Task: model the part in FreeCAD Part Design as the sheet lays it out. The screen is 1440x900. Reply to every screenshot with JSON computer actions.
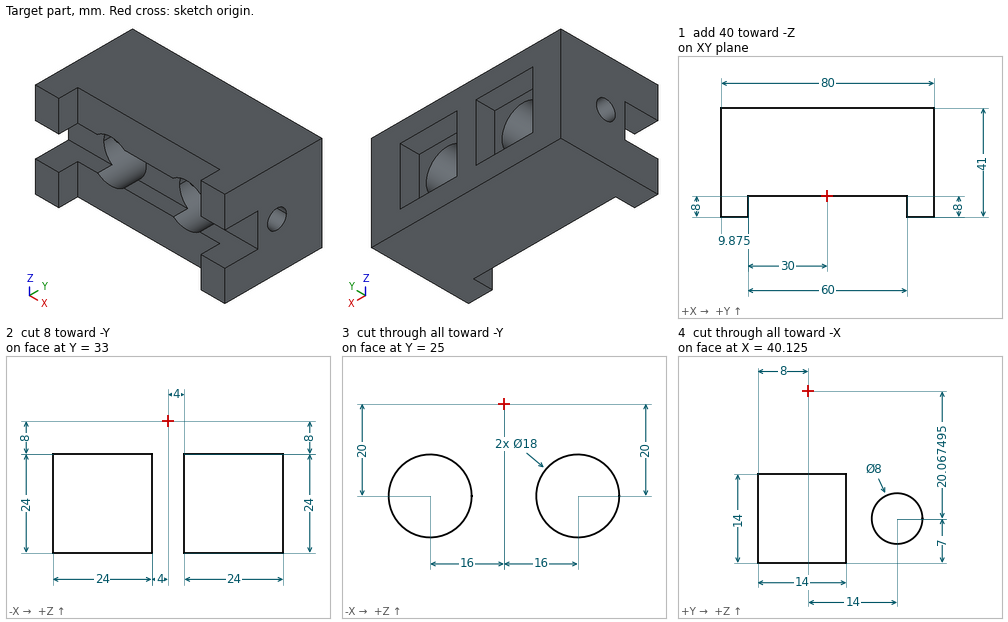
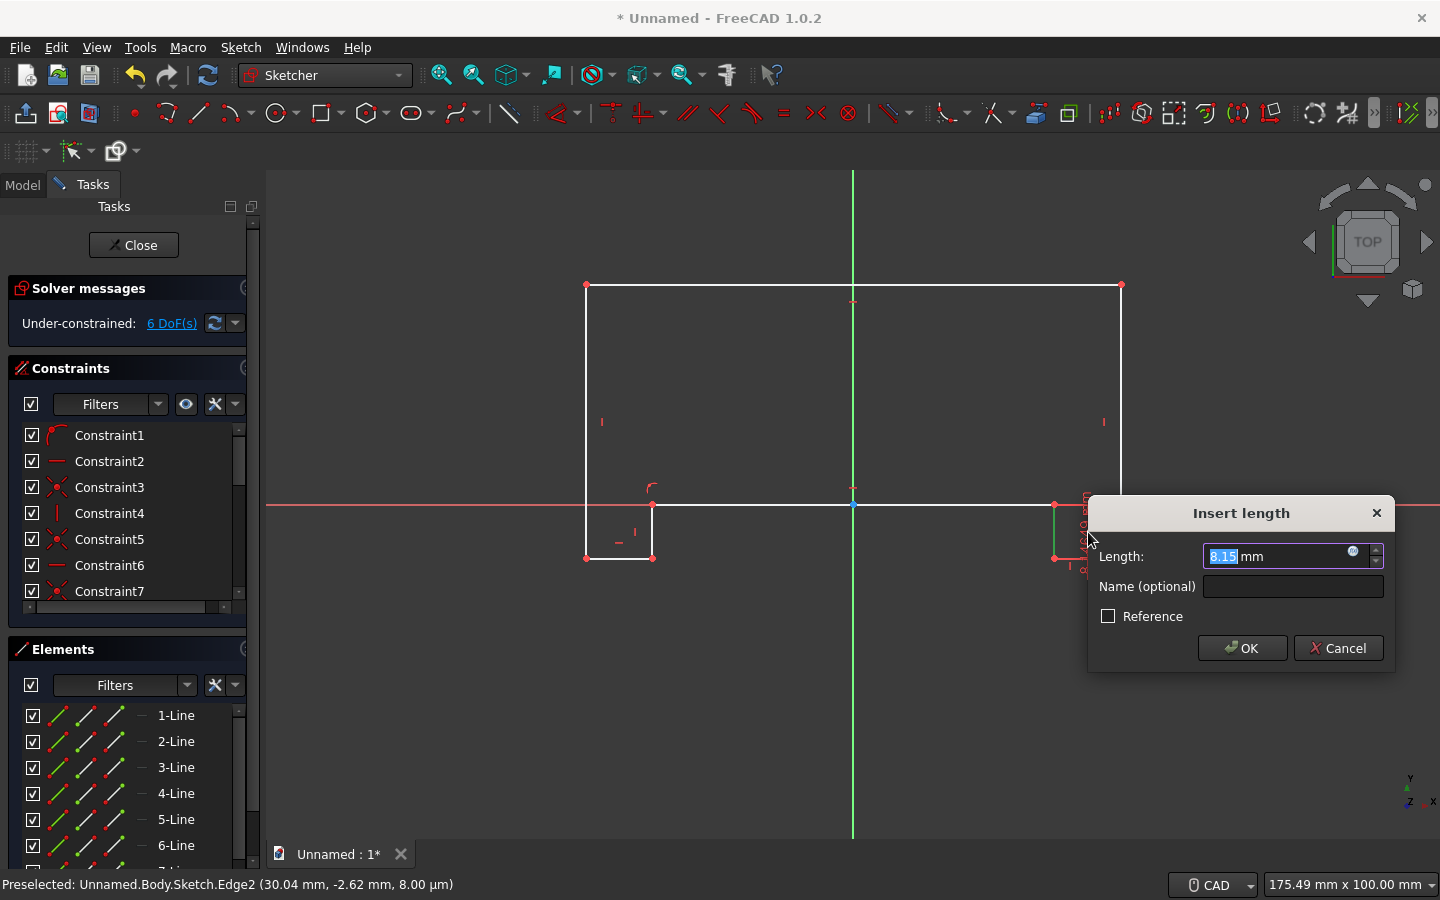
{"action": "type", "text": "8"}
{"action": "key", "text": "Return"}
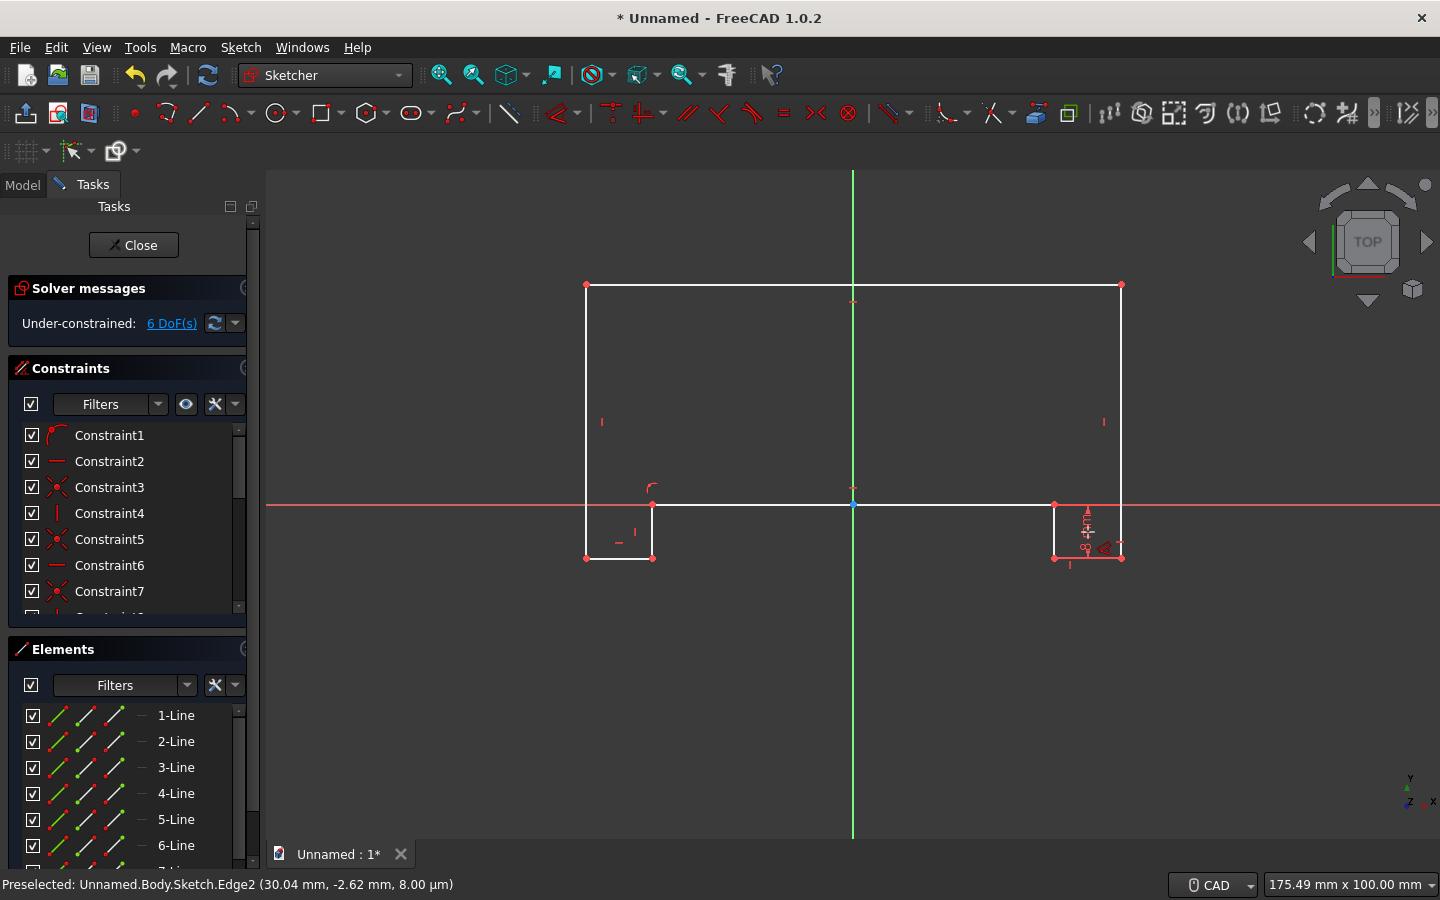
{"action": "left_click", "coordinate": [652, 543]}
{"action": "left_click", "coordinate": [618, 532]}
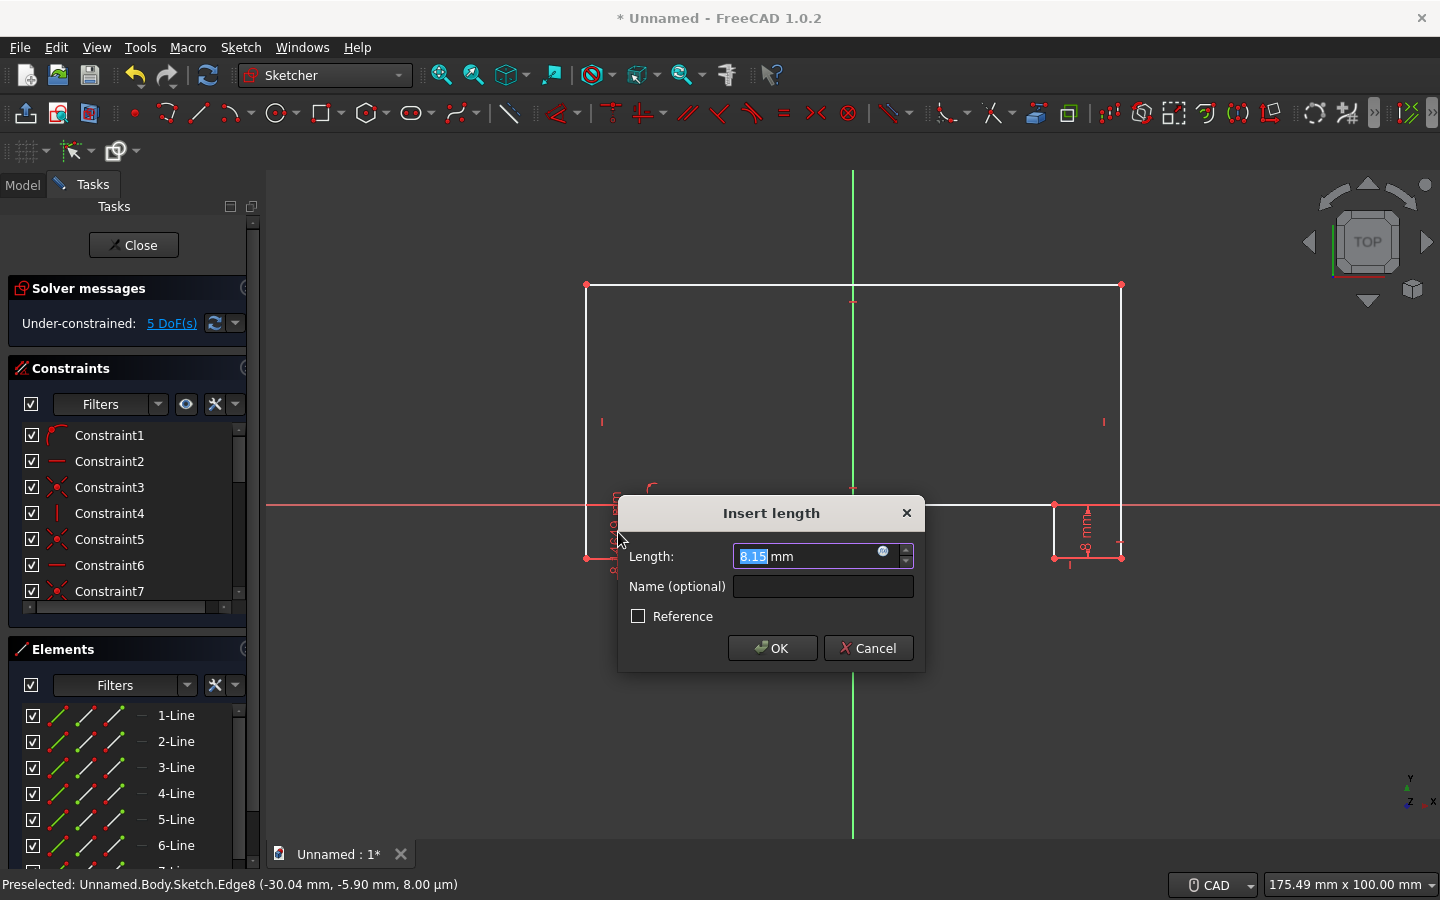
{"action": "type", "text": "8"}
{"action": "key", "text": "Return"}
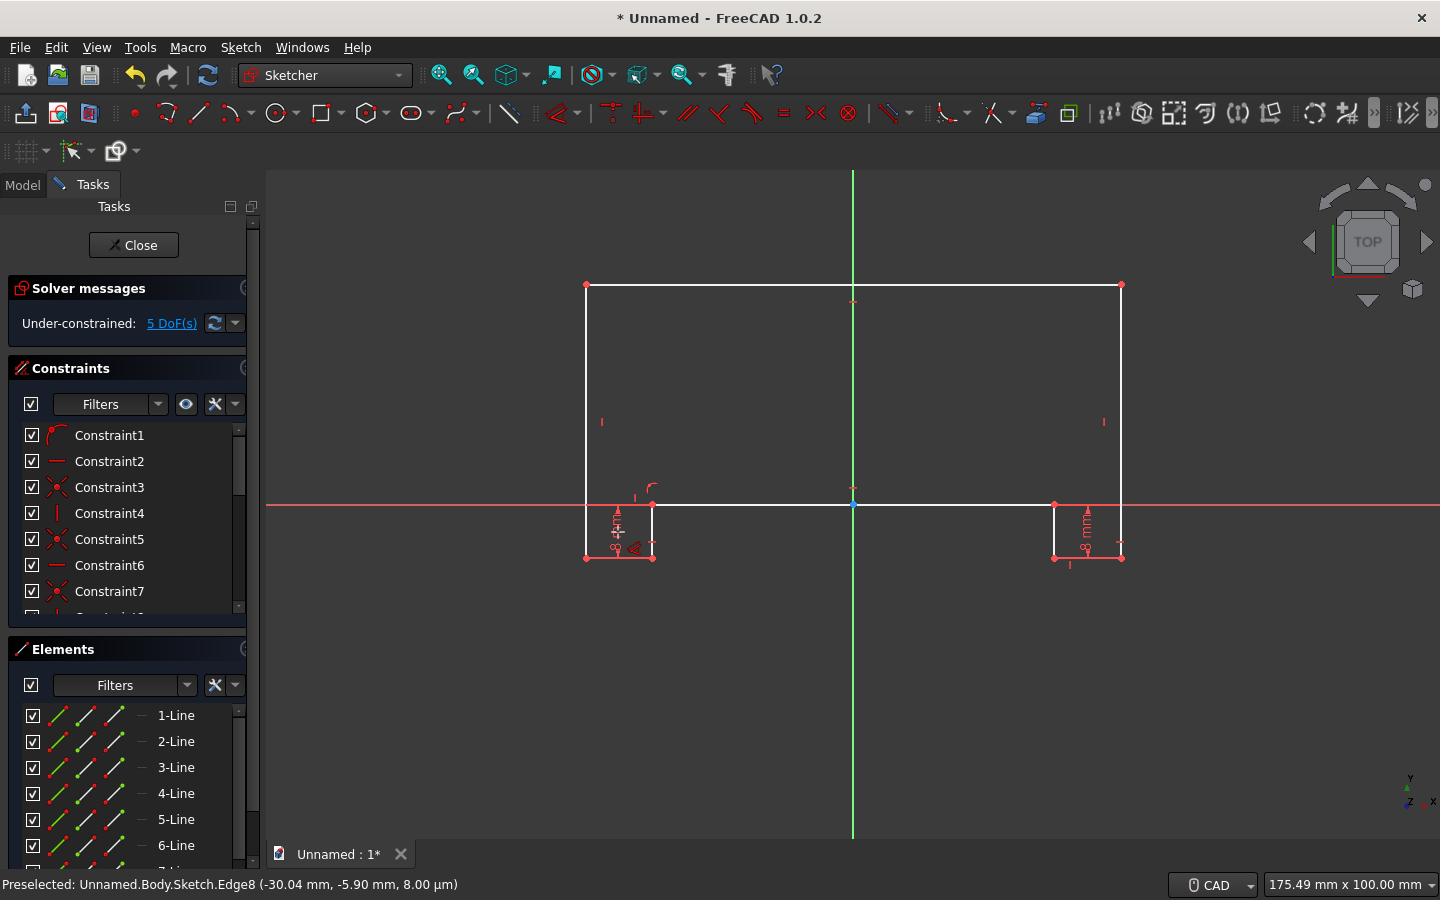
{"action": "left_click", "coordinate": [773, 504]}
{"action": "left_click", "coordinate": [761, 538]}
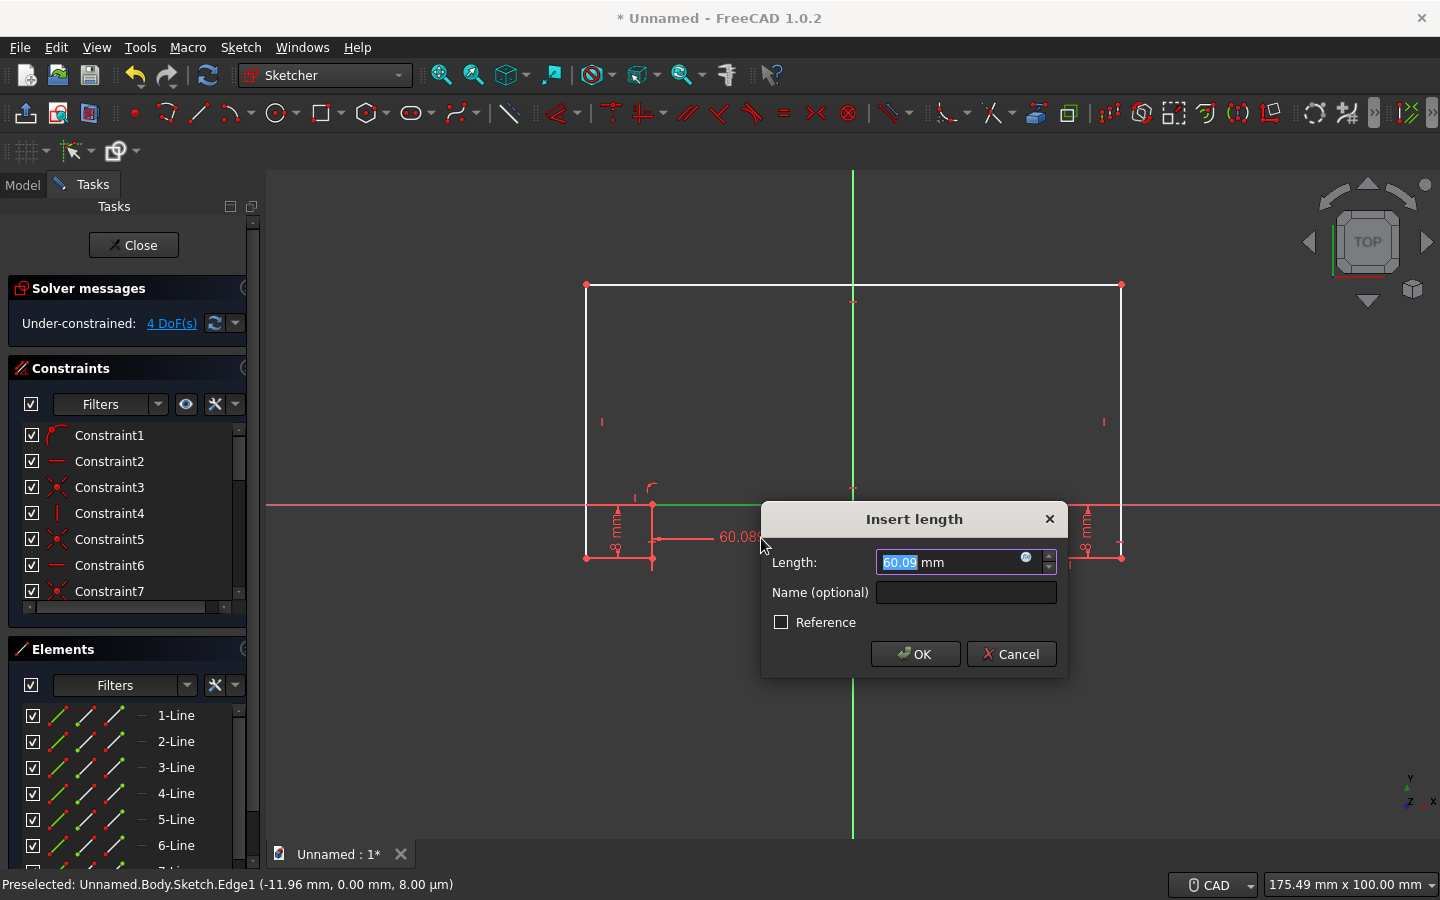
{"action": "type", "text": "60"}
{"action": "key", "text": "Return"}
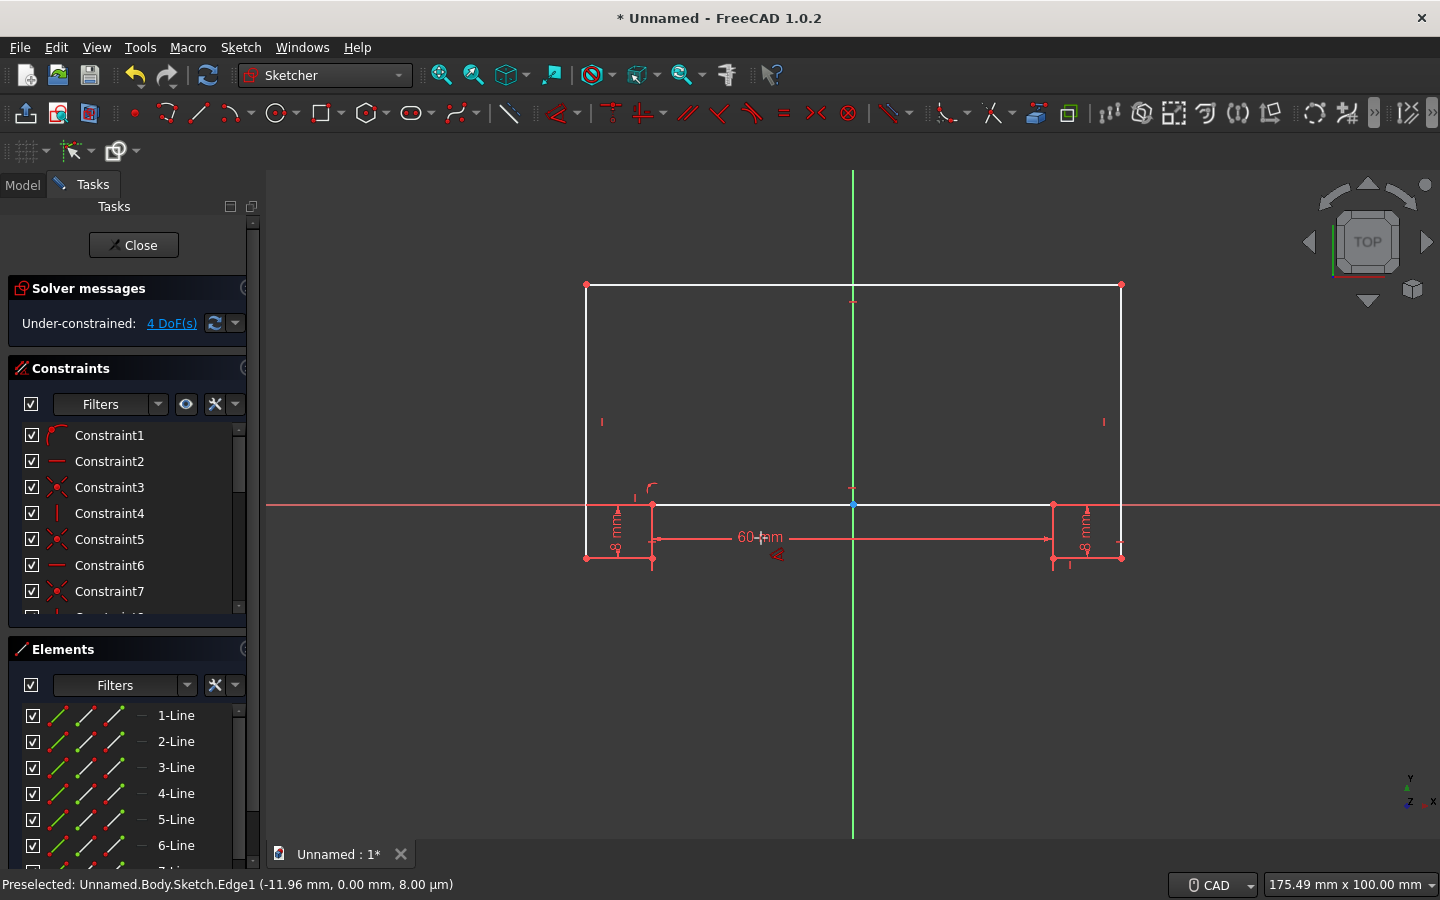
{"action": "left_click", "coordinate": [1121, 476]}
{"action": "left_click", "coordinate": [1155, 422]}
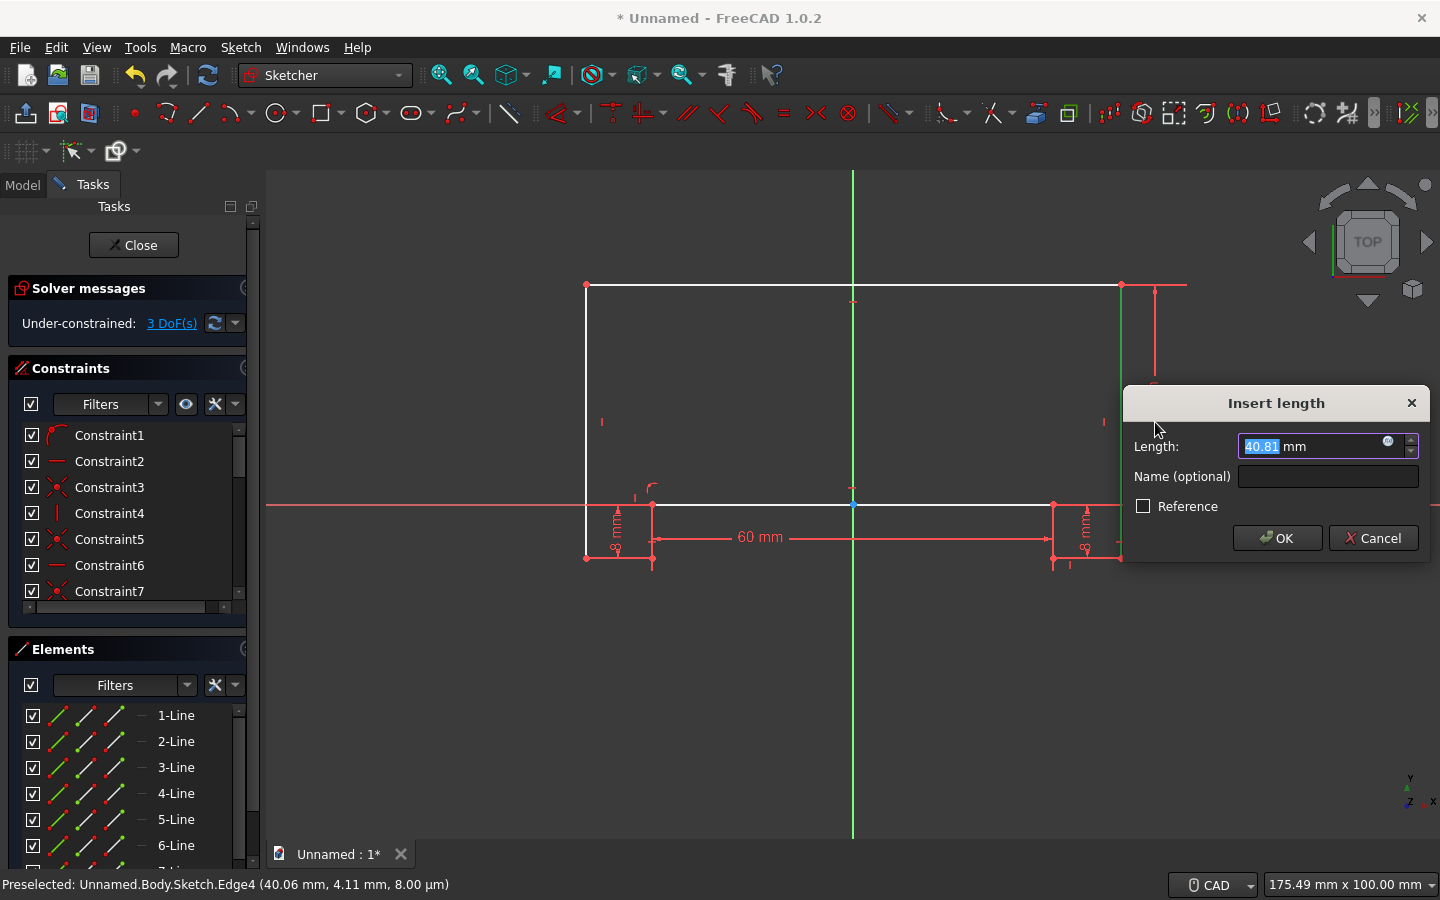
{"action": "type", "text": "41"}
{"action": "key", "text": "Return"}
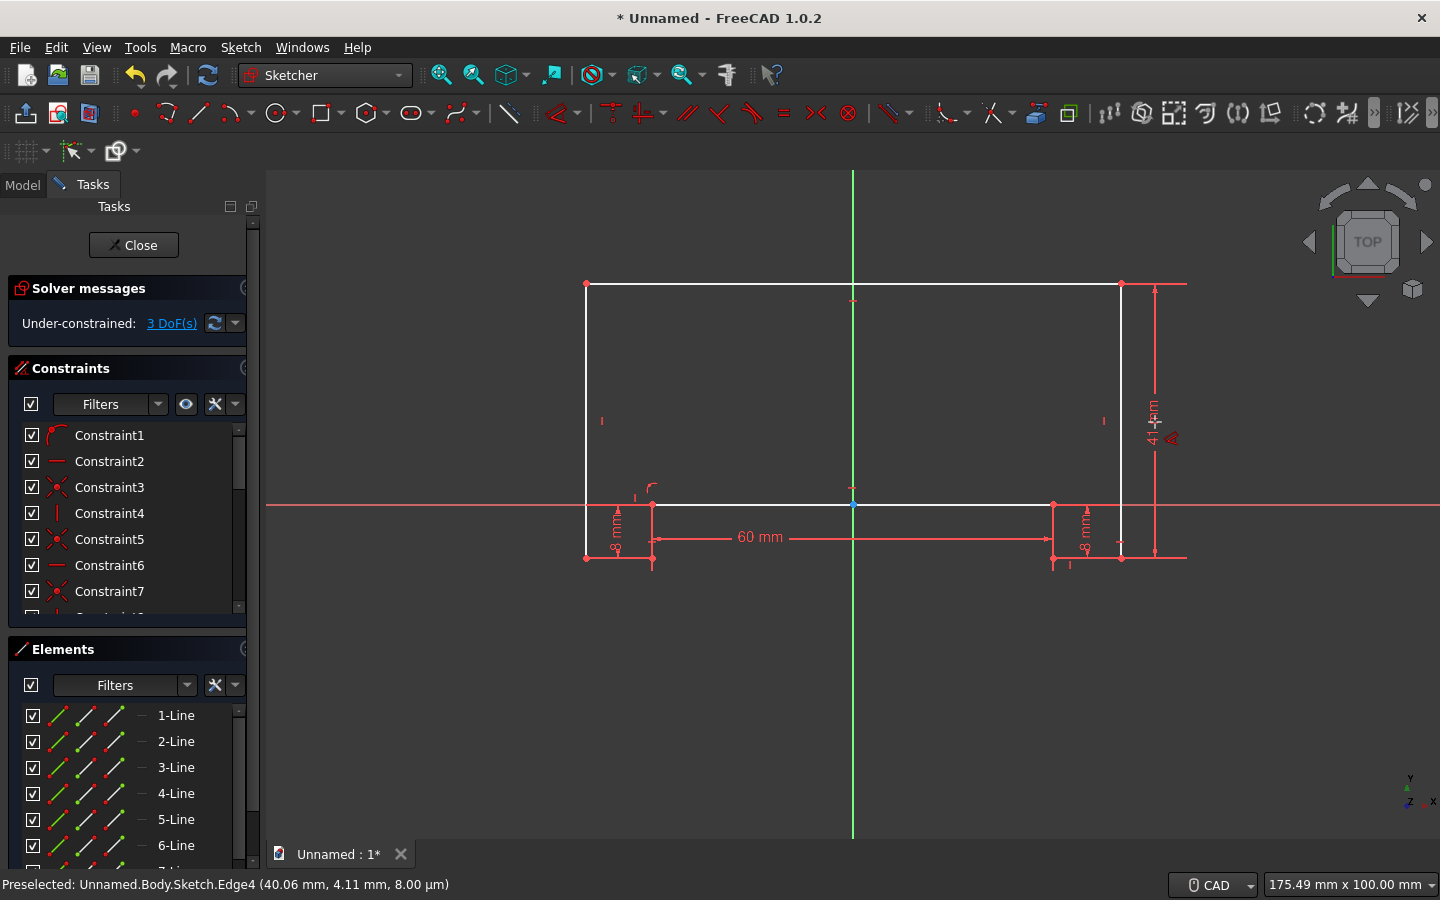
{"action": "left_click", "coordinate": [961, 284]}
{"action": "left_click", "coordinate": [730, 250]}